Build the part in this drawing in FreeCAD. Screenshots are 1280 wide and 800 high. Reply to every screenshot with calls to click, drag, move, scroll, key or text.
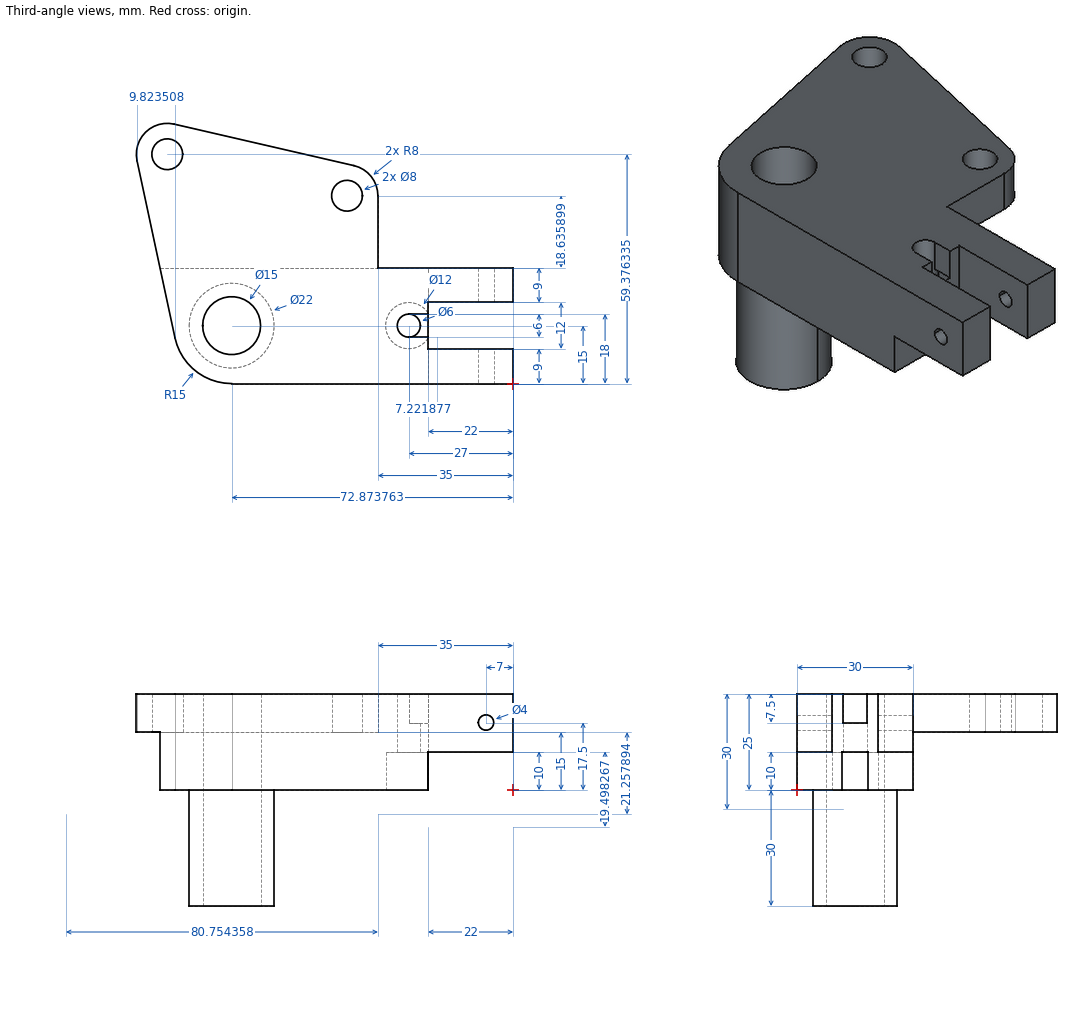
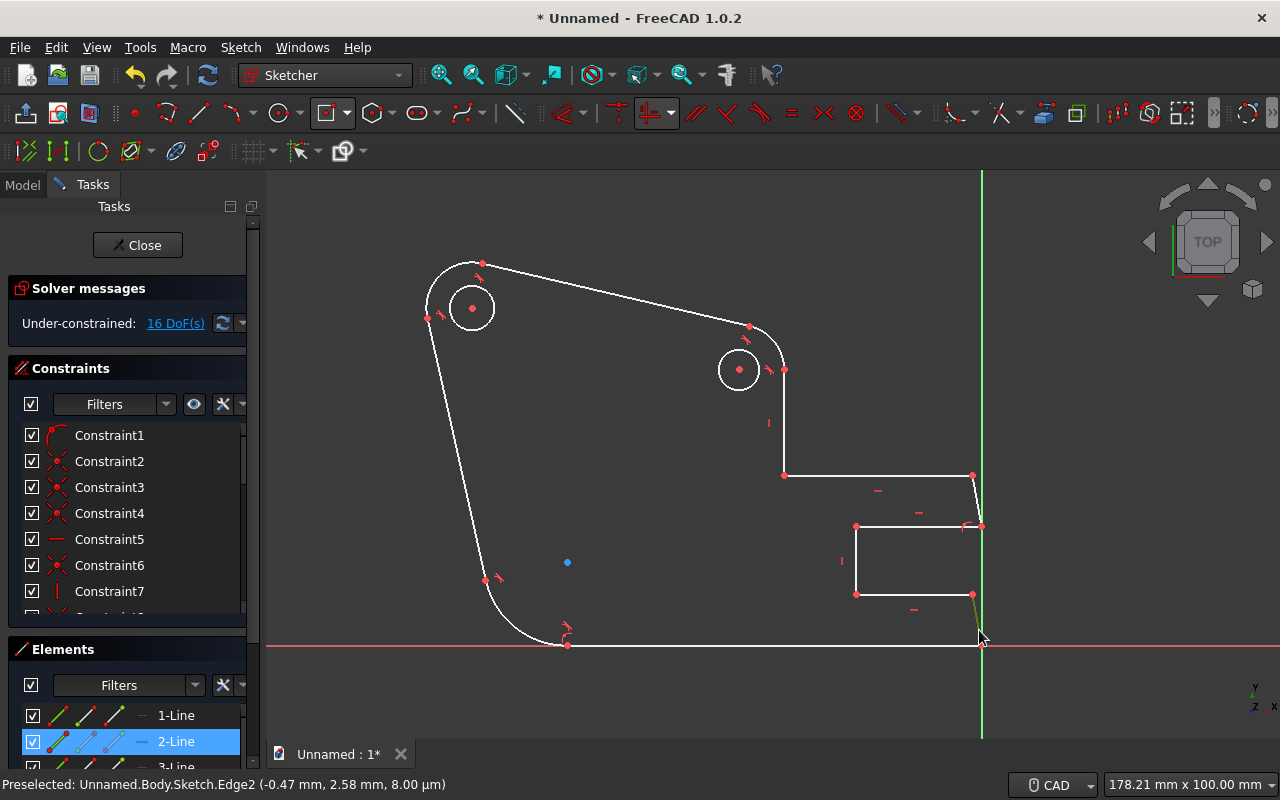
click(674, 114)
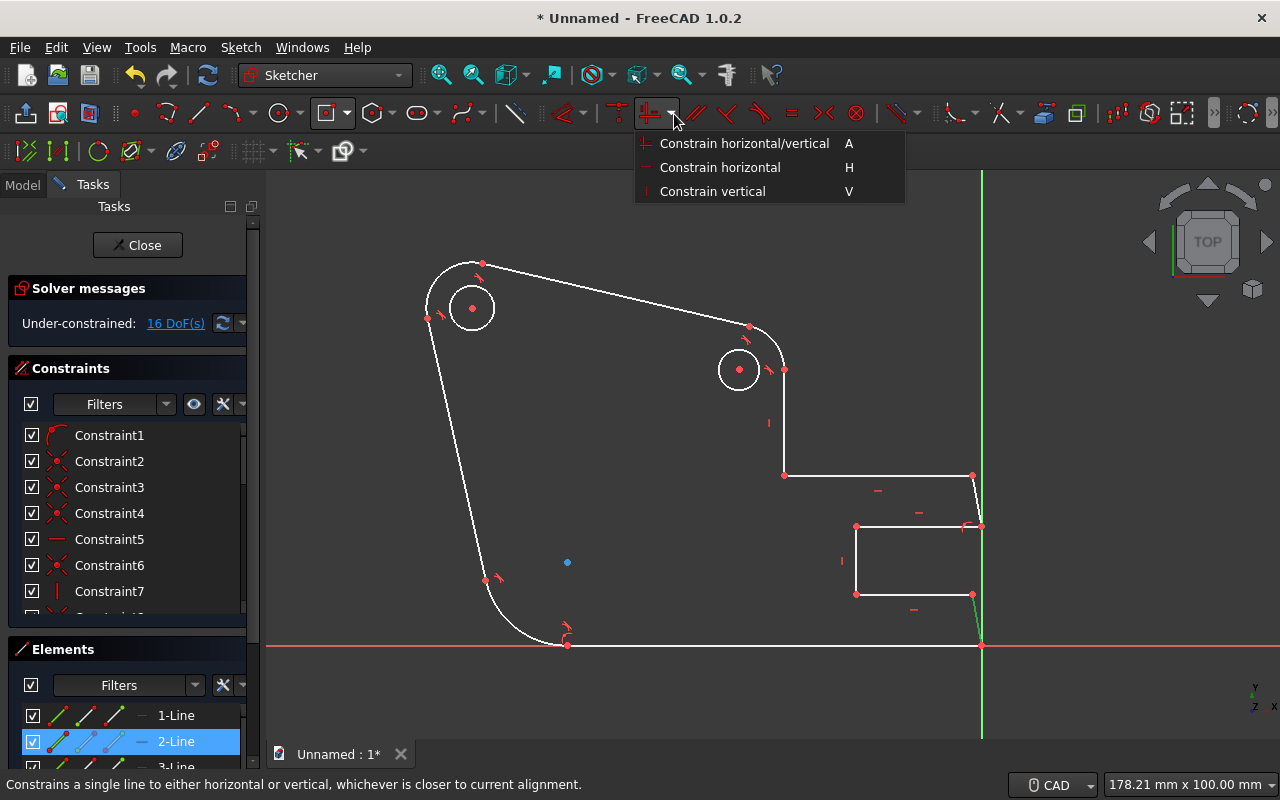
click(770, 191)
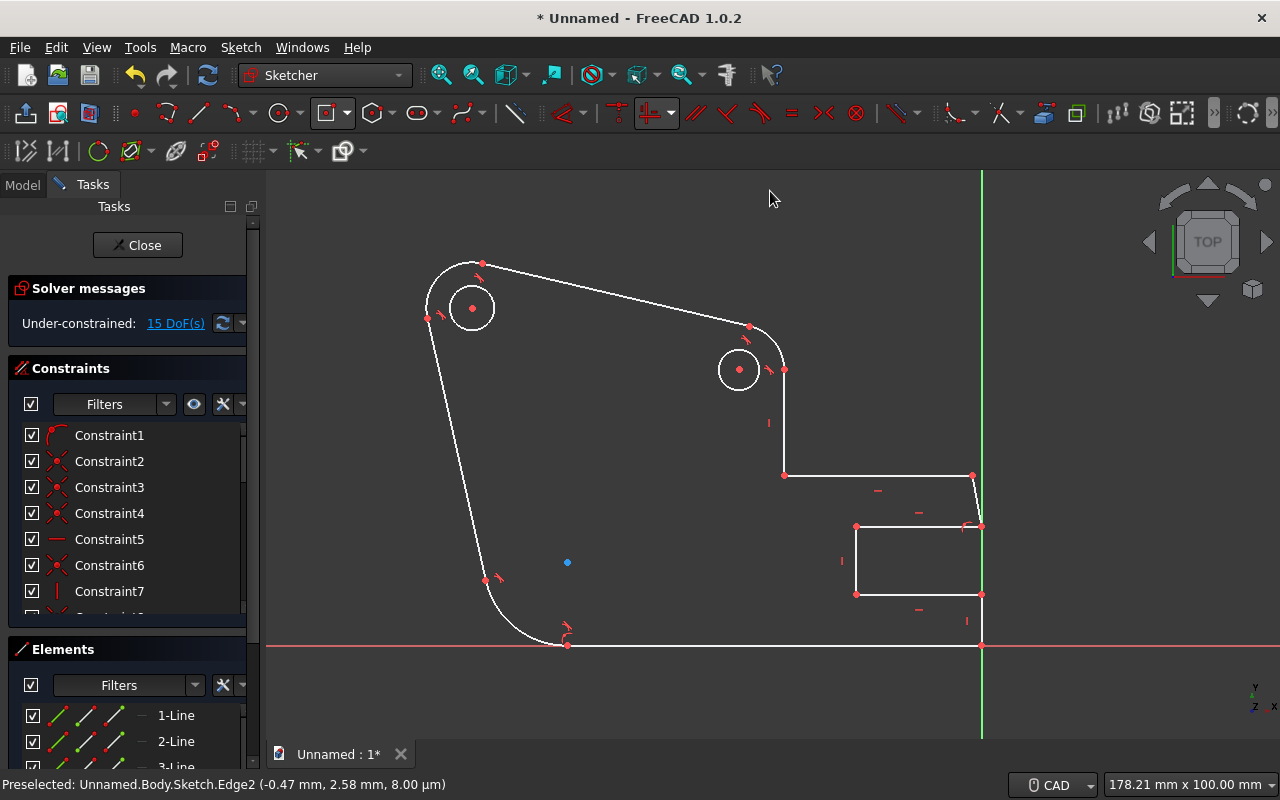
click(979, 512)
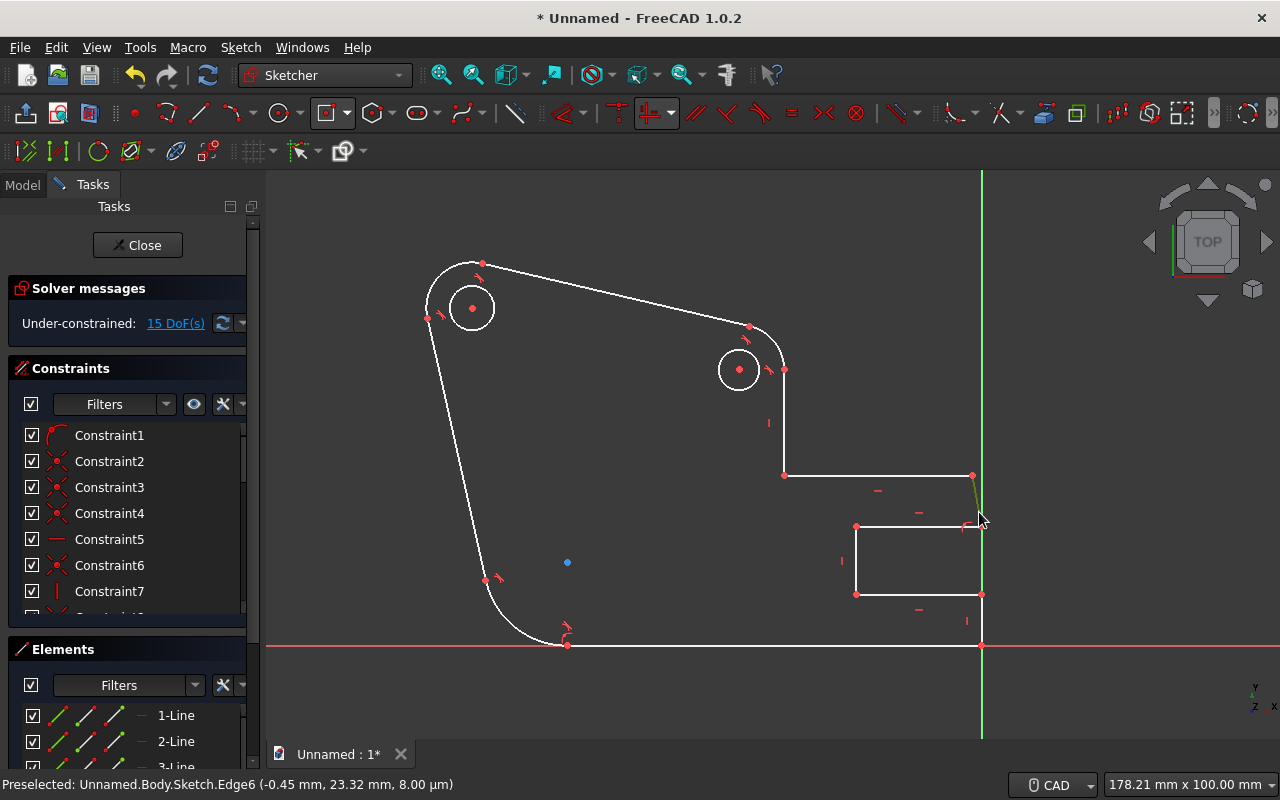
key(v)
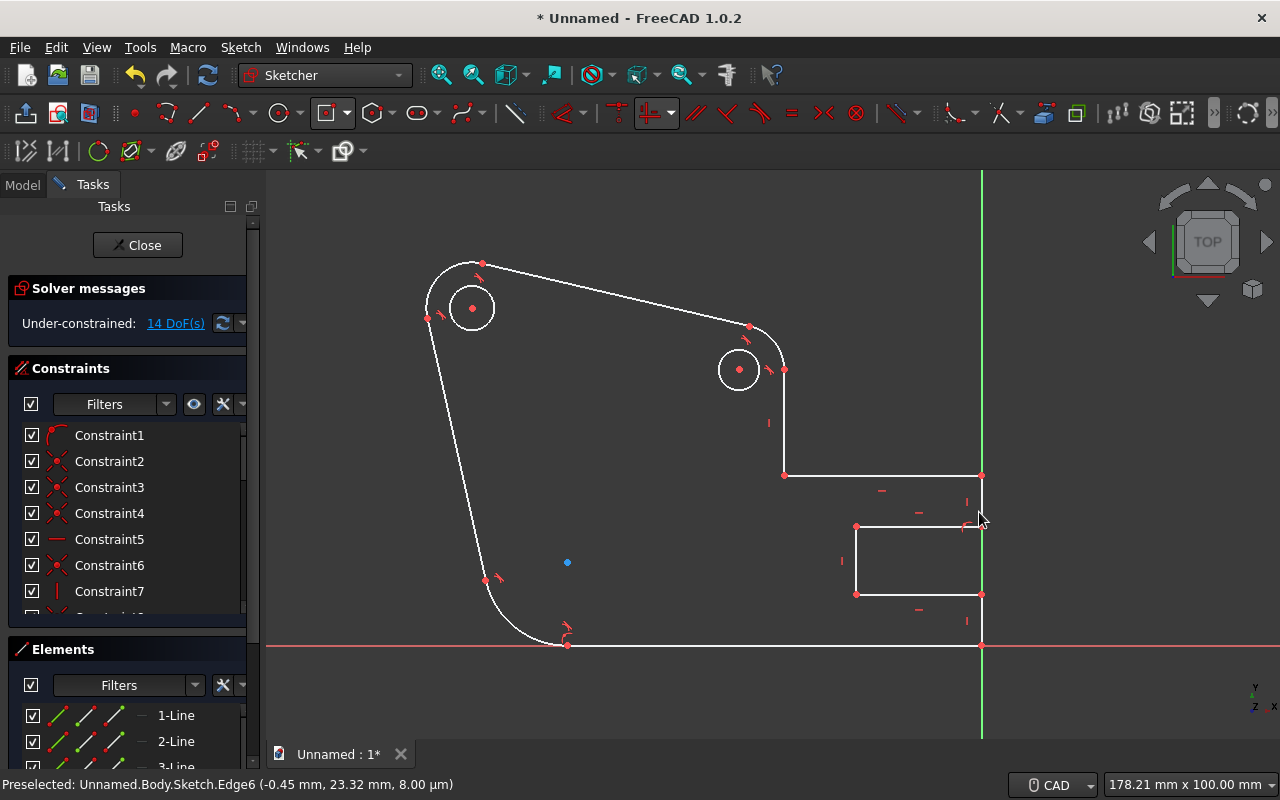
click(781, 352)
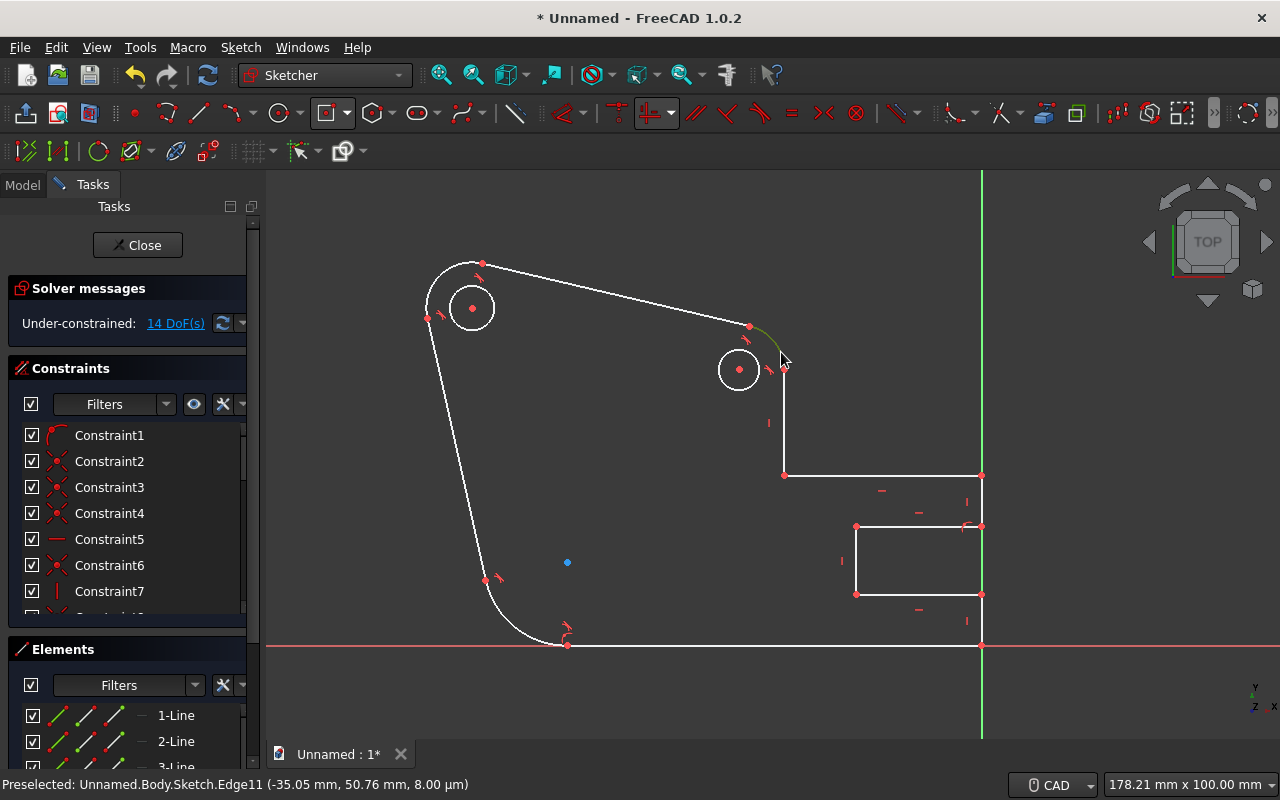
click(455, 266)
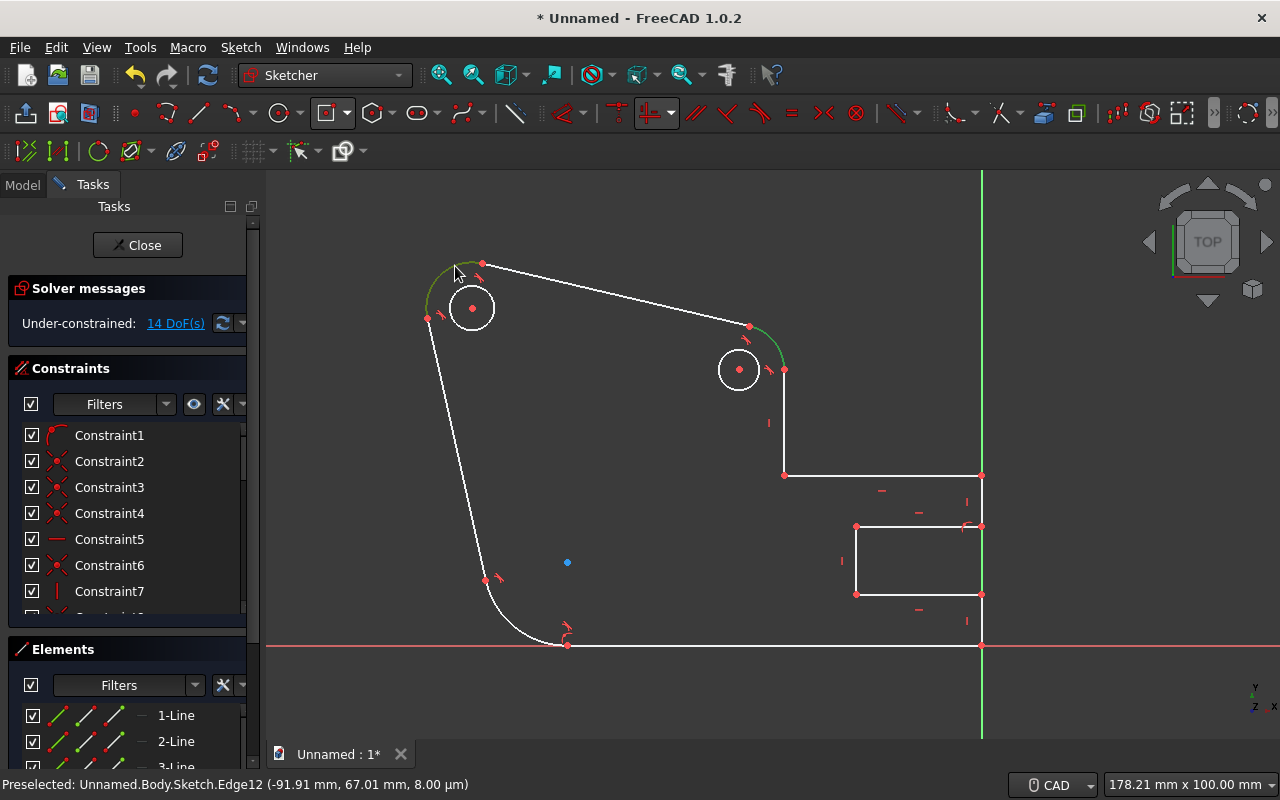
click(792, 114)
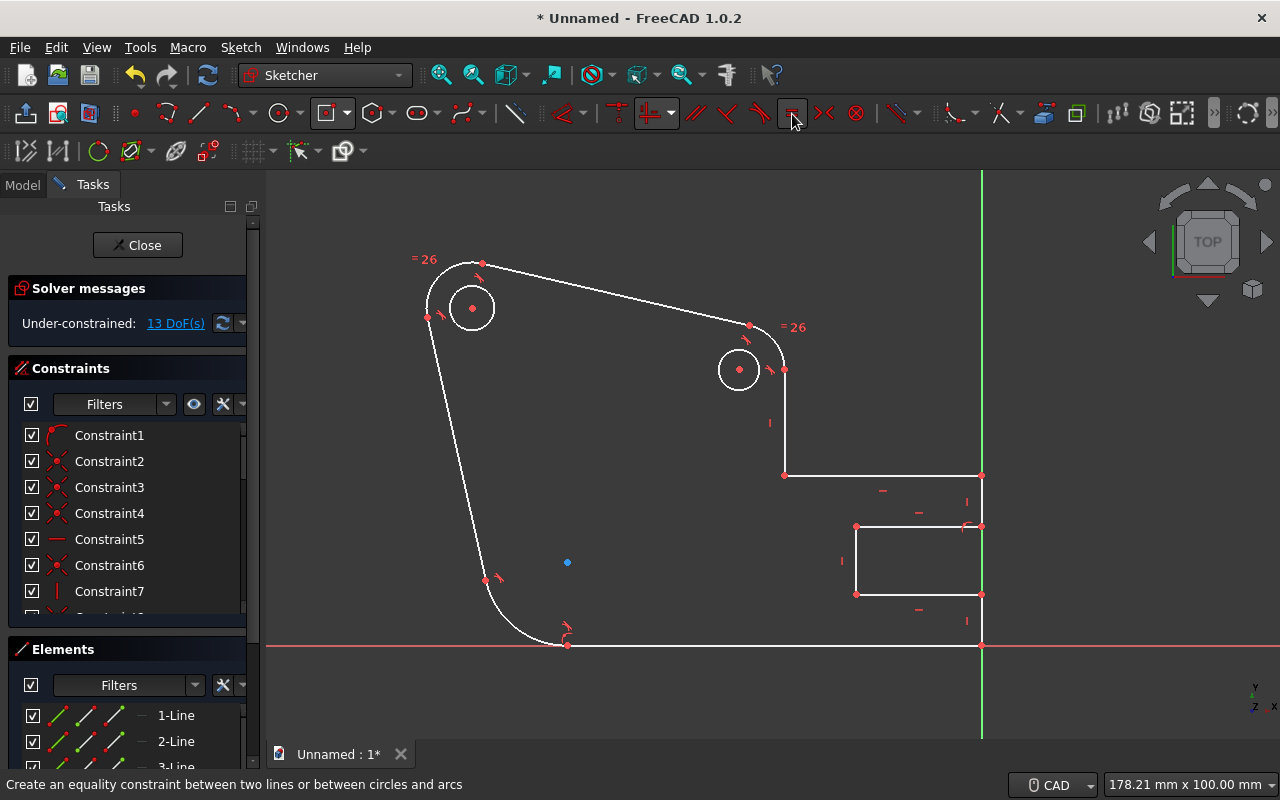
click(753, 356)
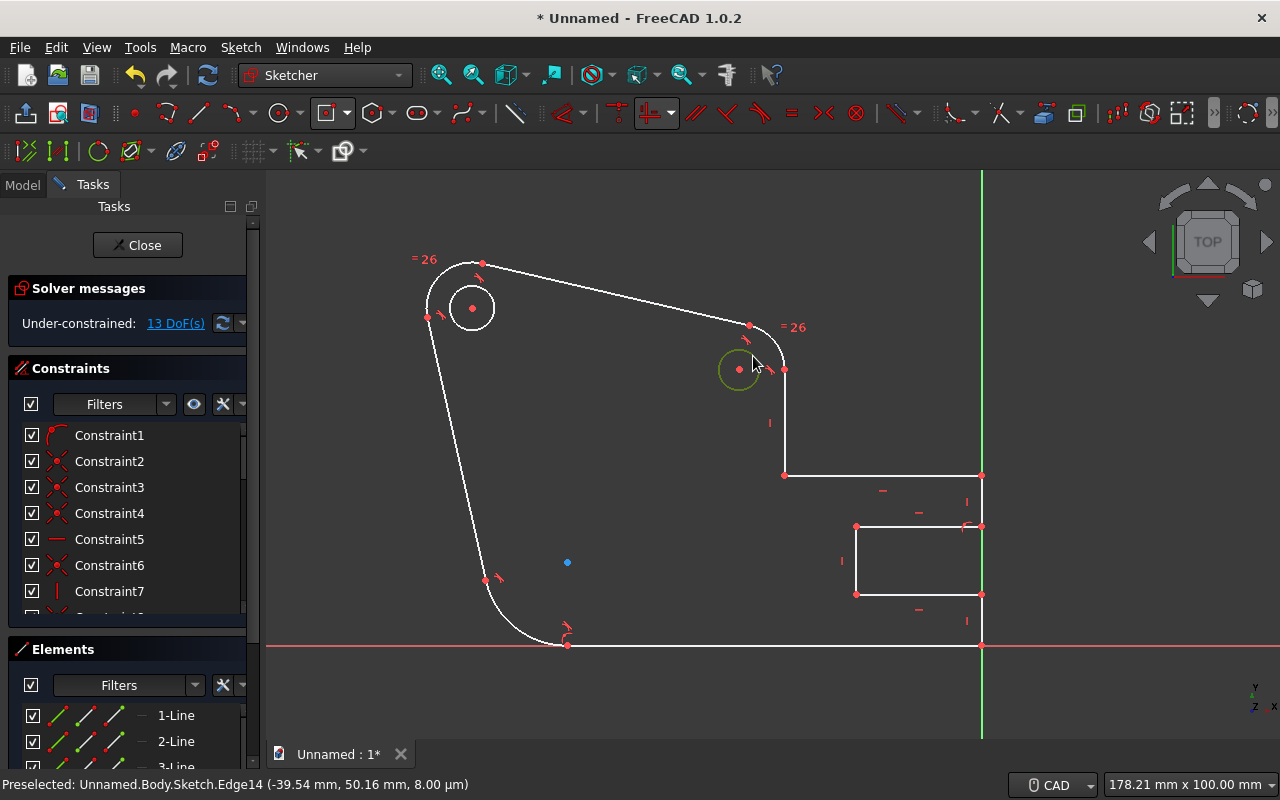
click(488, 292)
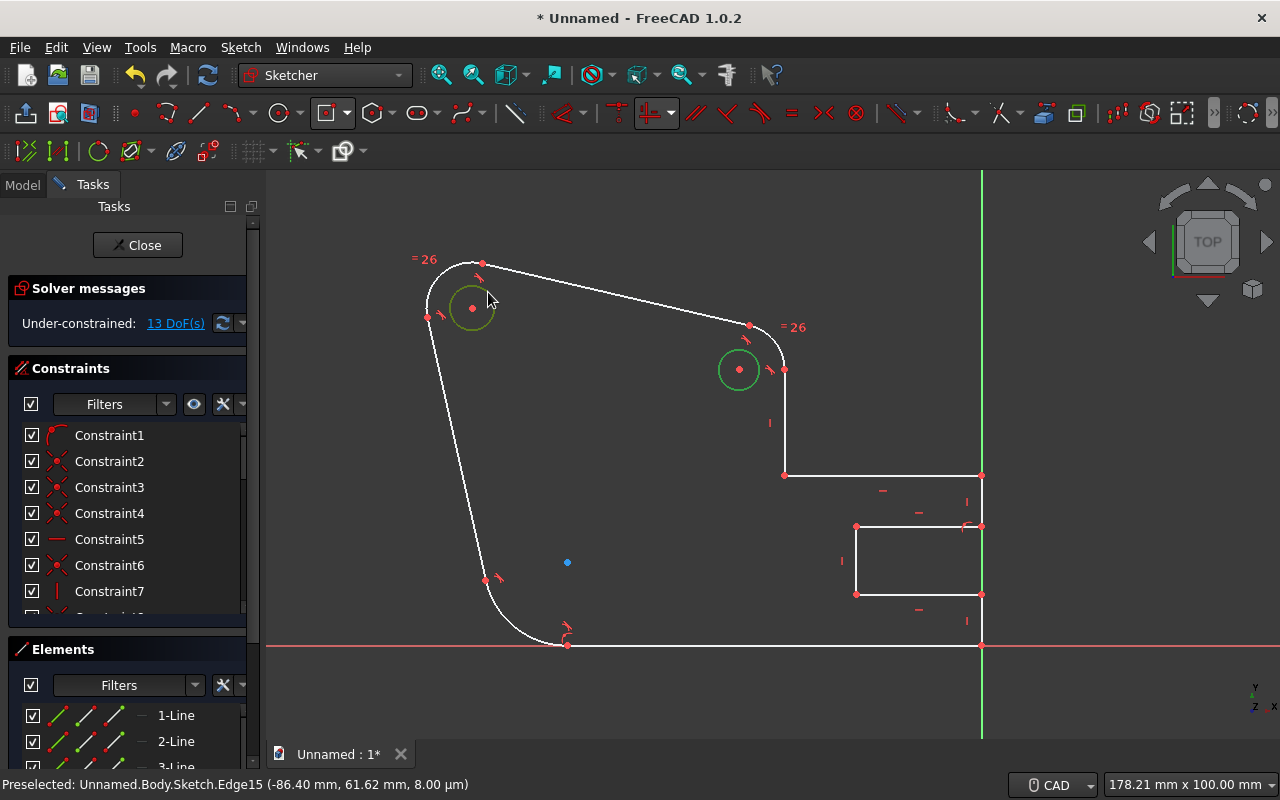
click(792, 114)